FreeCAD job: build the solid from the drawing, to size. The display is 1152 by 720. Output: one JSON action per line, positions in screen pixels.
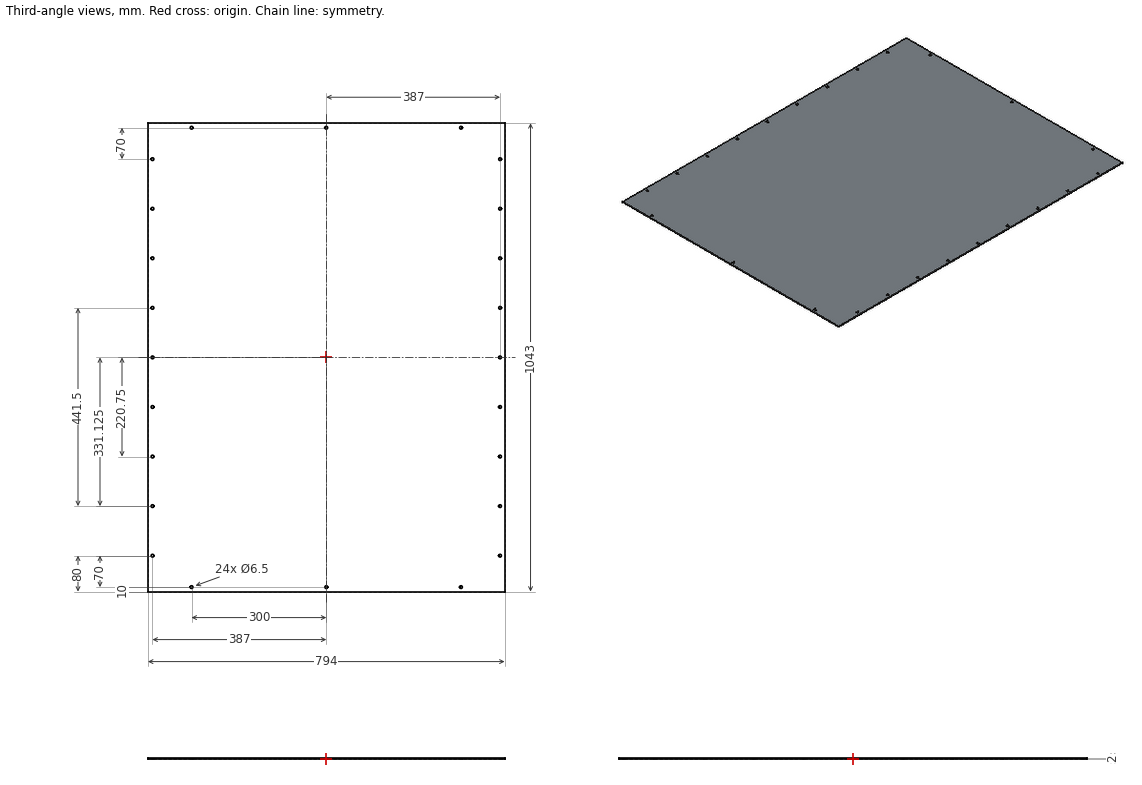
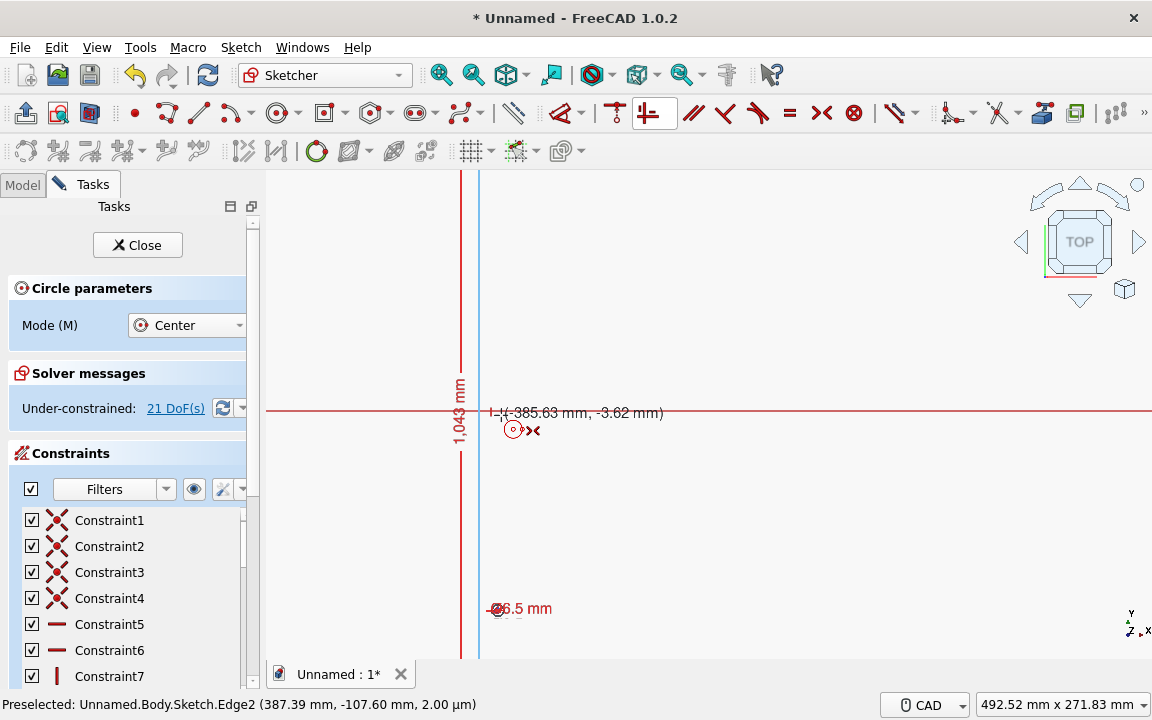
{"action": "left_click", "coordinate": [497, 411]}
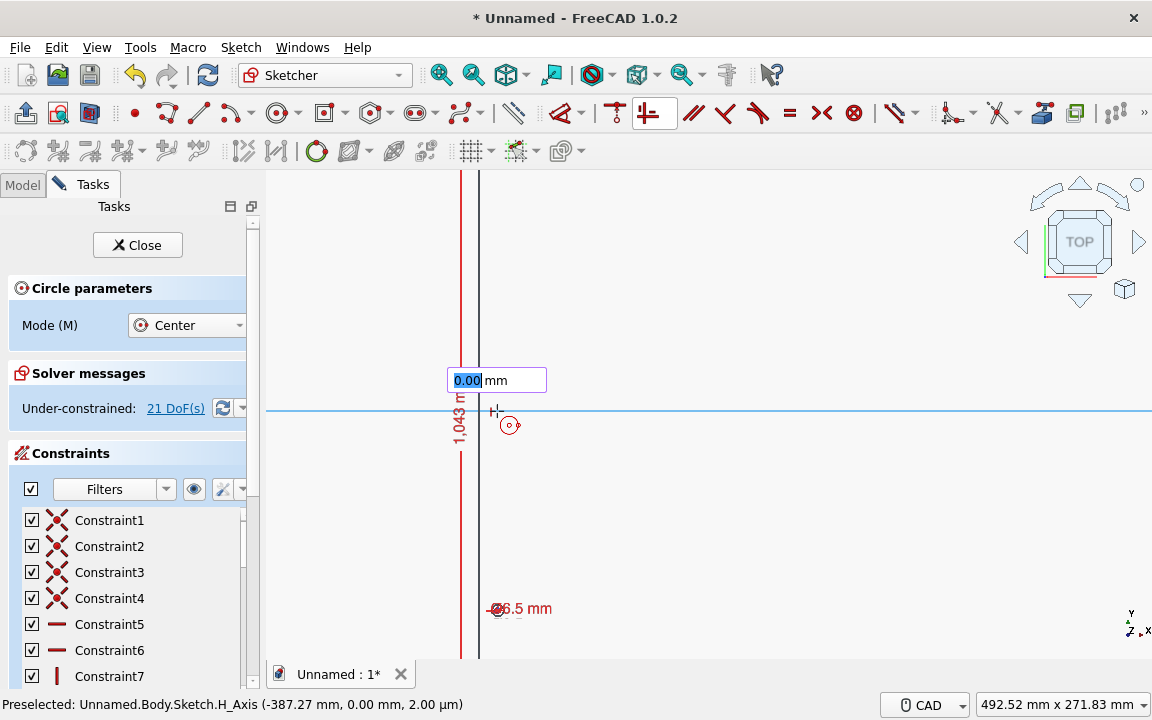
{"action": "scroll", "coordinate": [495, 417], "scroll_direction": "up", "scroll_amount": 6}
{"action": "mouse_move", "coordinate": [496, 416]}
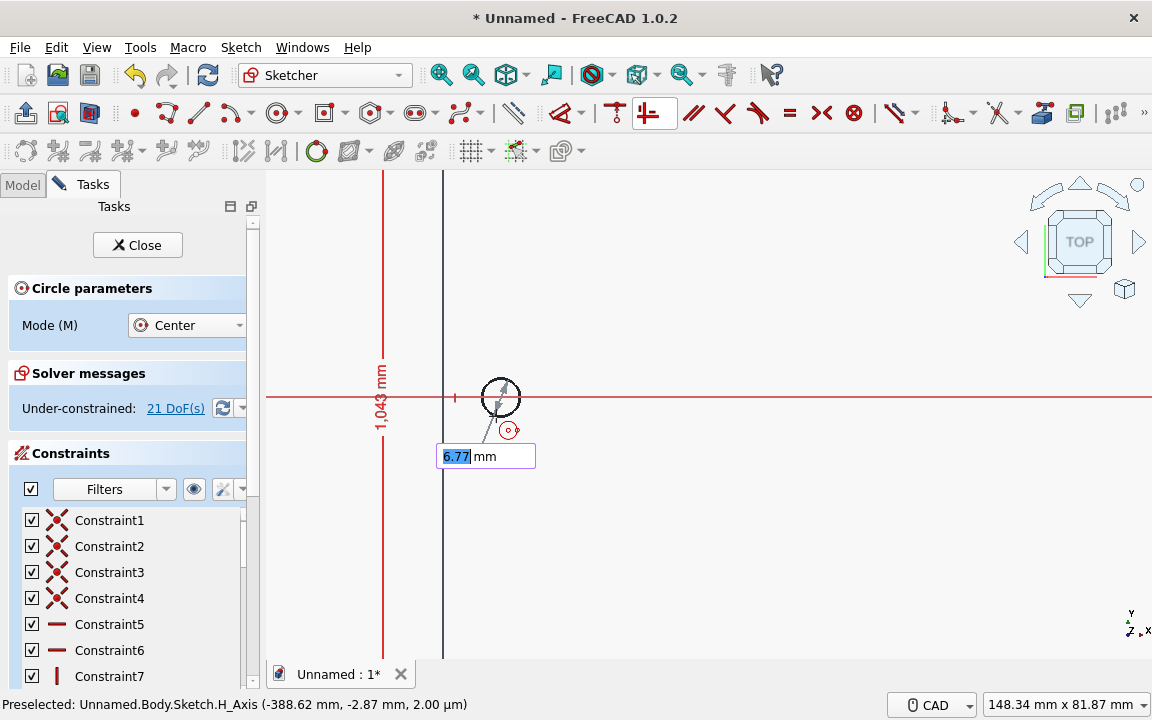
{"action": "type", "text": "6.5"}
{"action": "key", "text": "Return"}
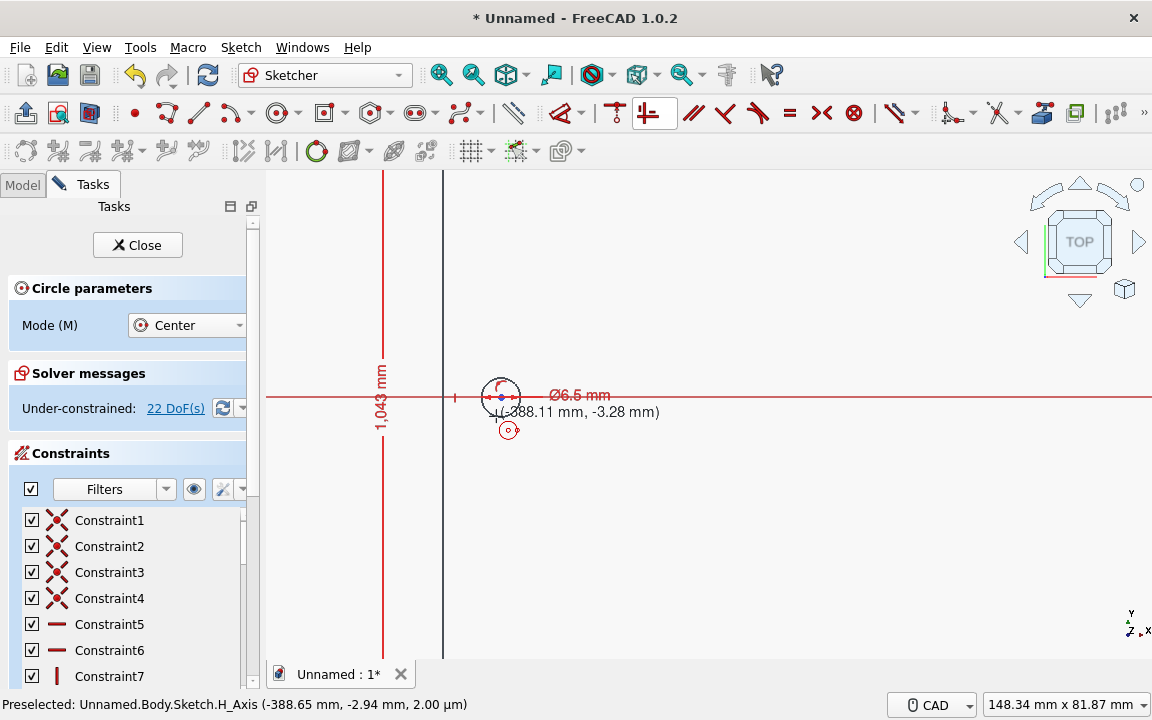
{"action": "scroll", "coordinate": [527, 415], "scroll_direction": "down", "scroll_amount": 15}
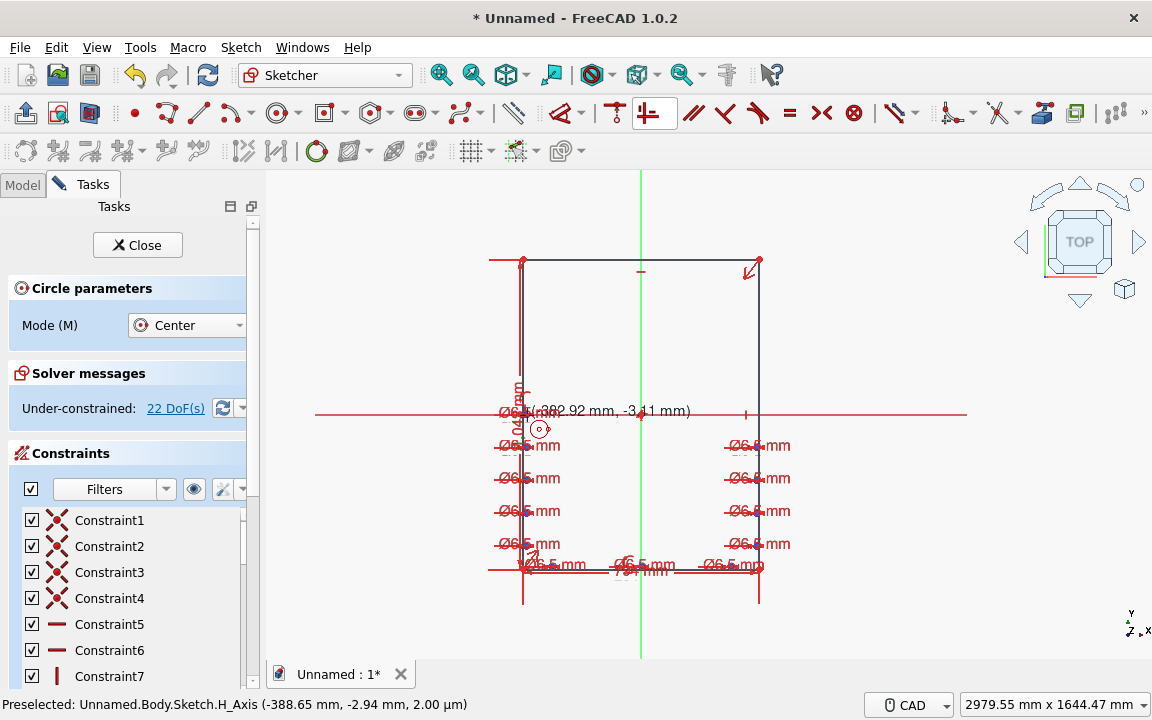
{"action": "scroll", "coordinate": [526, 382], "scroll_direction": "up", "scroll_amount": 16}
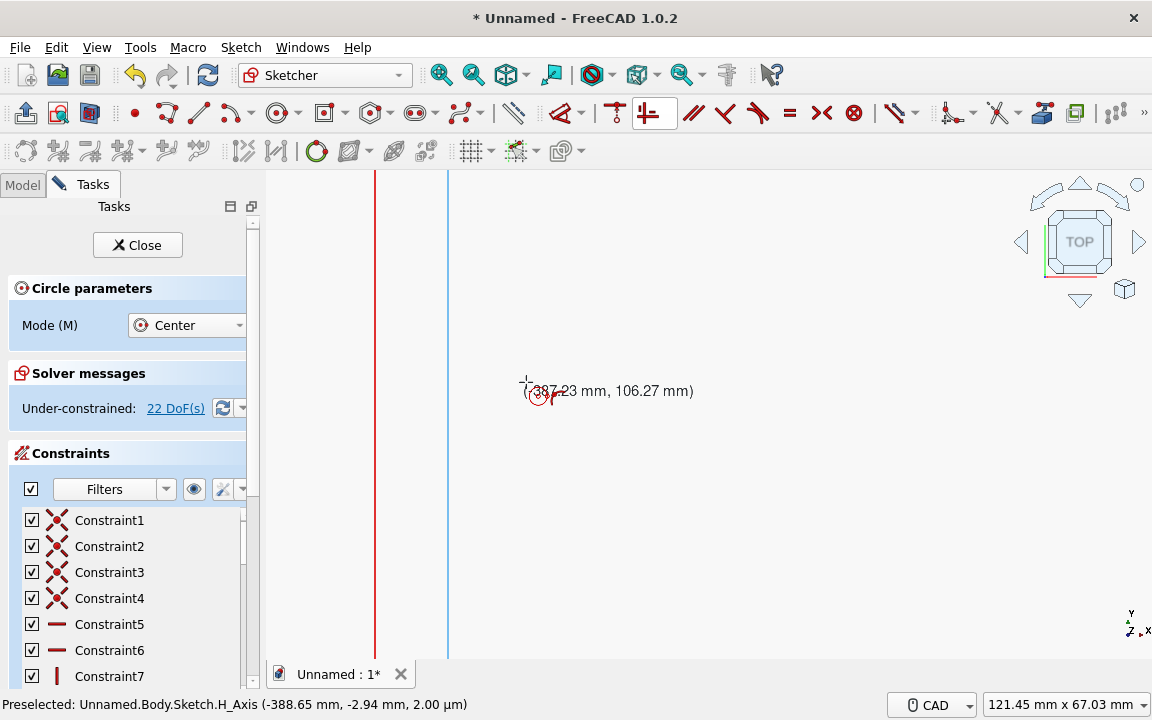
{"action": "scroll", "coordinate": [499, 375], "scroll_direction": "down", "scroll_amount": 15}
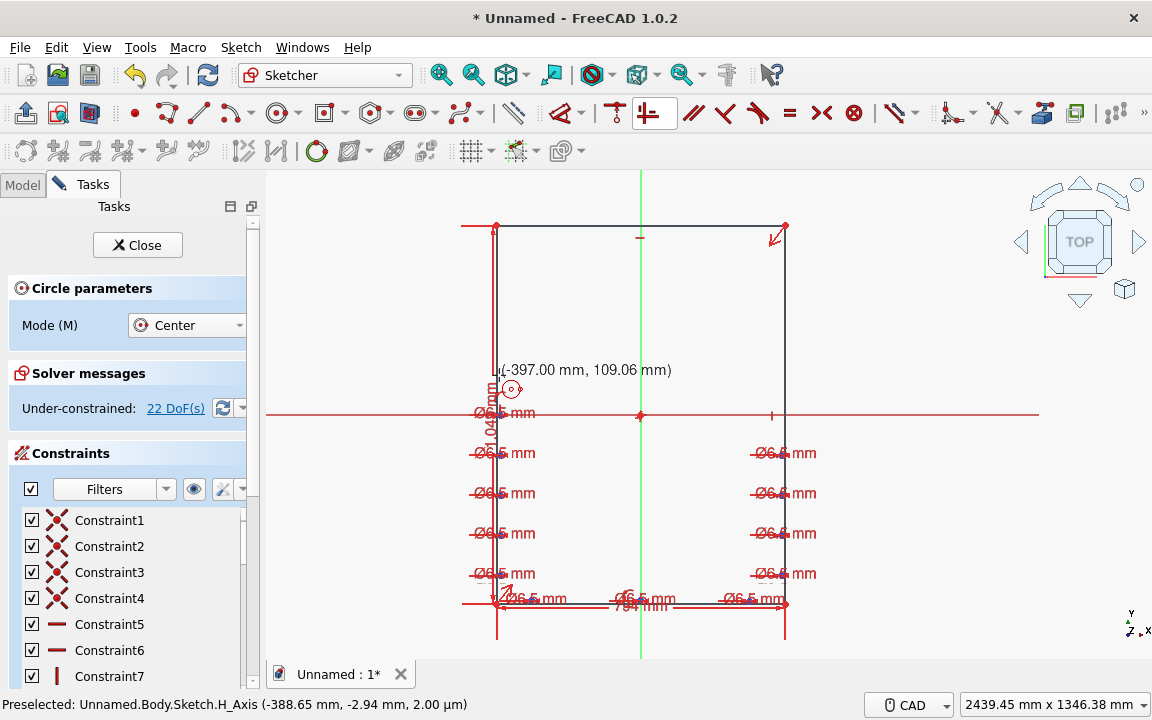
{"action": "scroll", "coordinate": [500, 375], "scroll_direction": "up", "scroll_amount": 8}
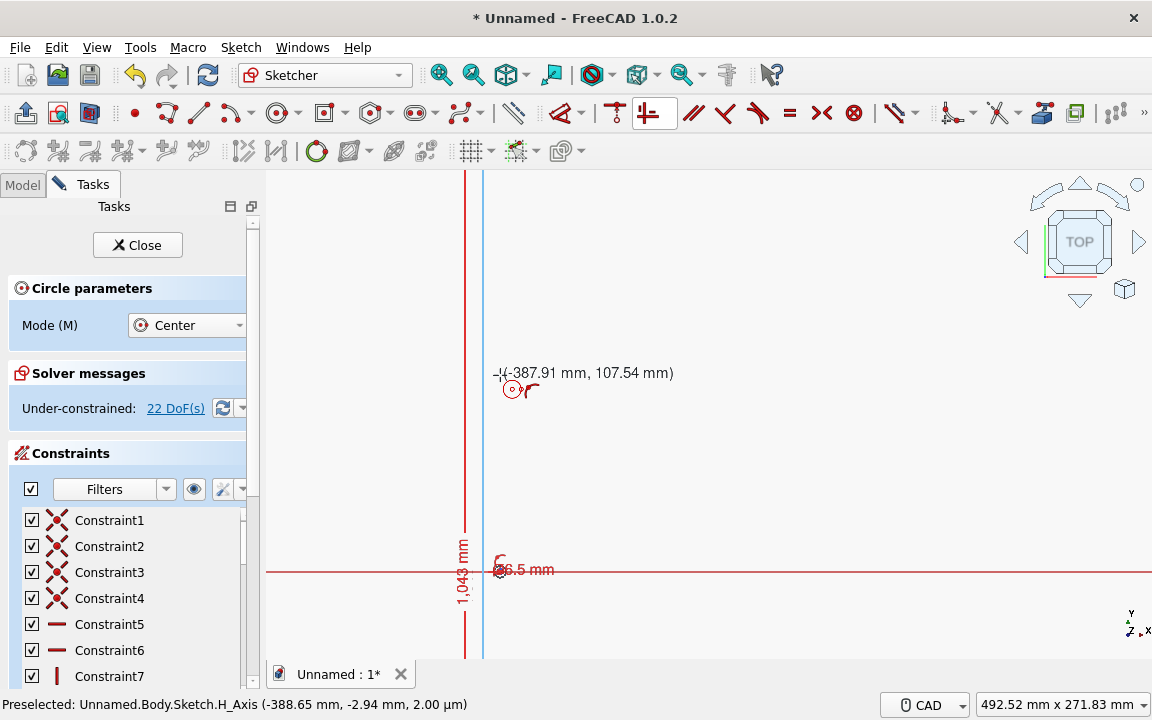
{"action": "left_click", "coordinate": [501, 373]}
{"action": "mouse_move", "coordinate": [505, 369]}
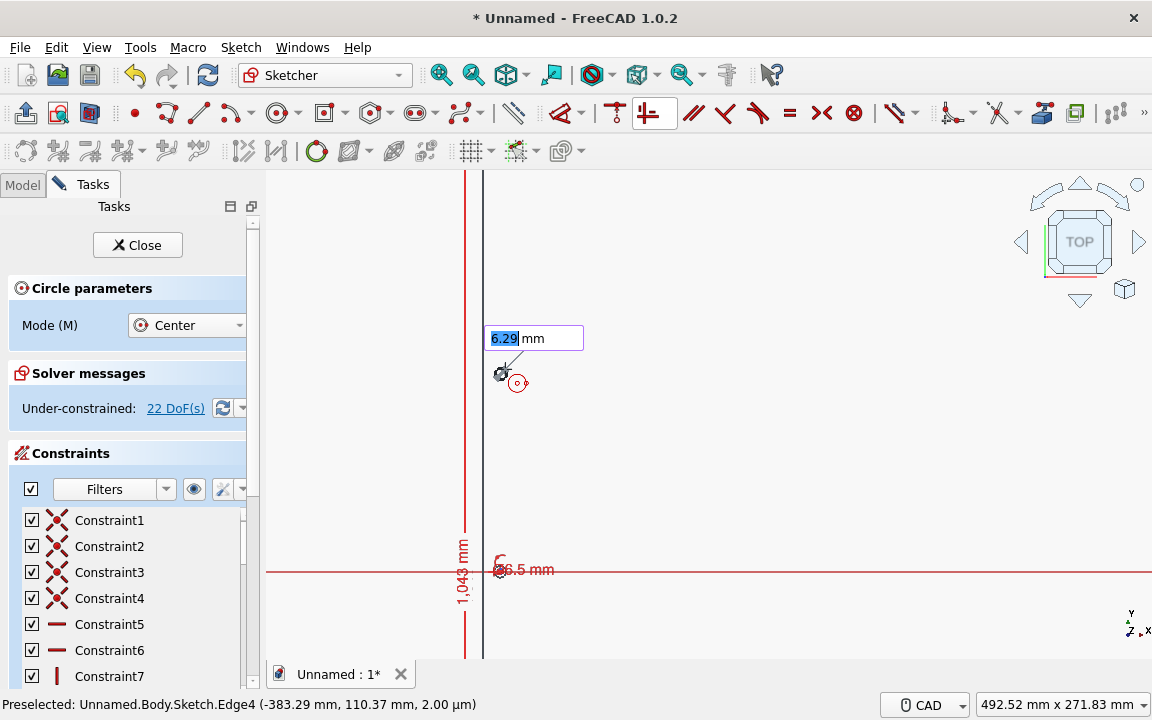
{"action": "type", "text": "6.5"}
{"action": "key", "text": "Return"}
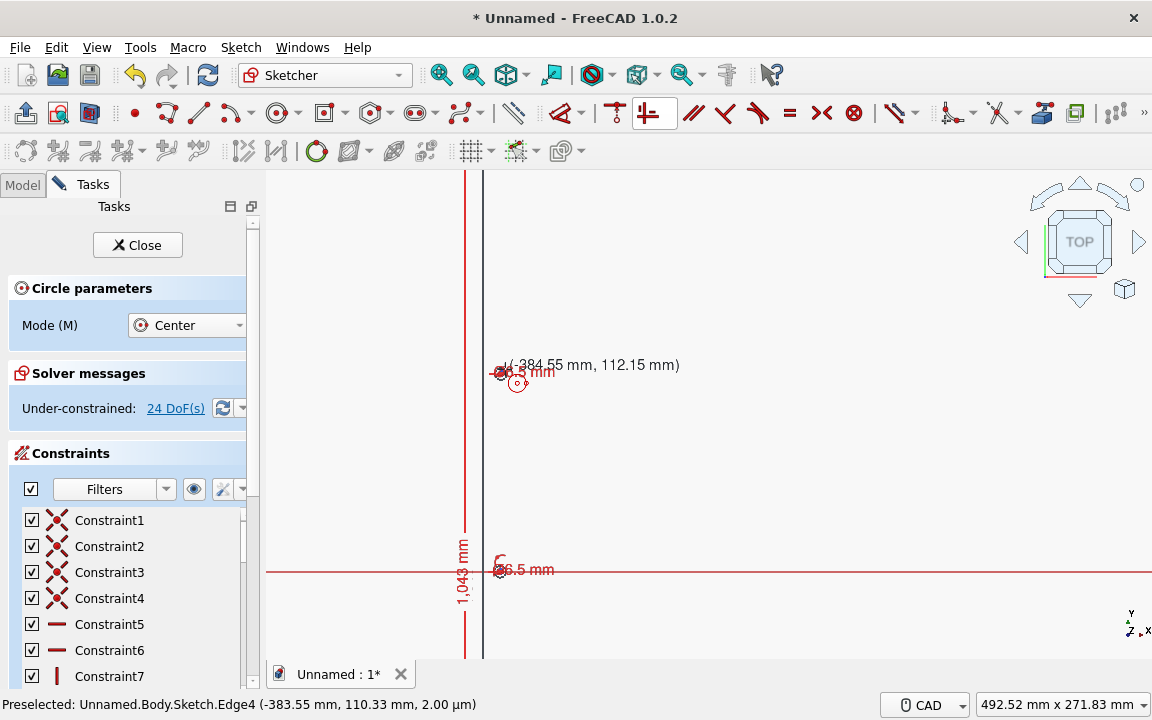
{"action": "scroll", "coordinate": [530, 383], "scroll_direction": "down", "scroll_amount": 9}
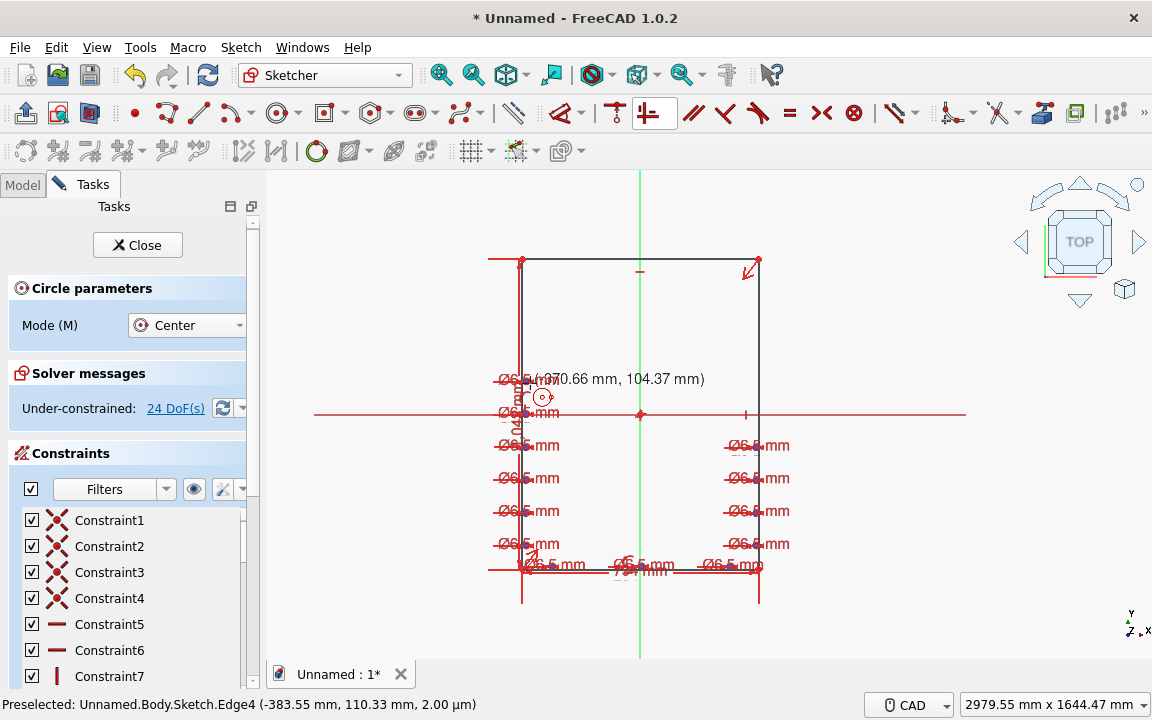
{"action": "scroll", "coordinate": [525, 349], "scroll_direction": "up", "scroll_amount": 16}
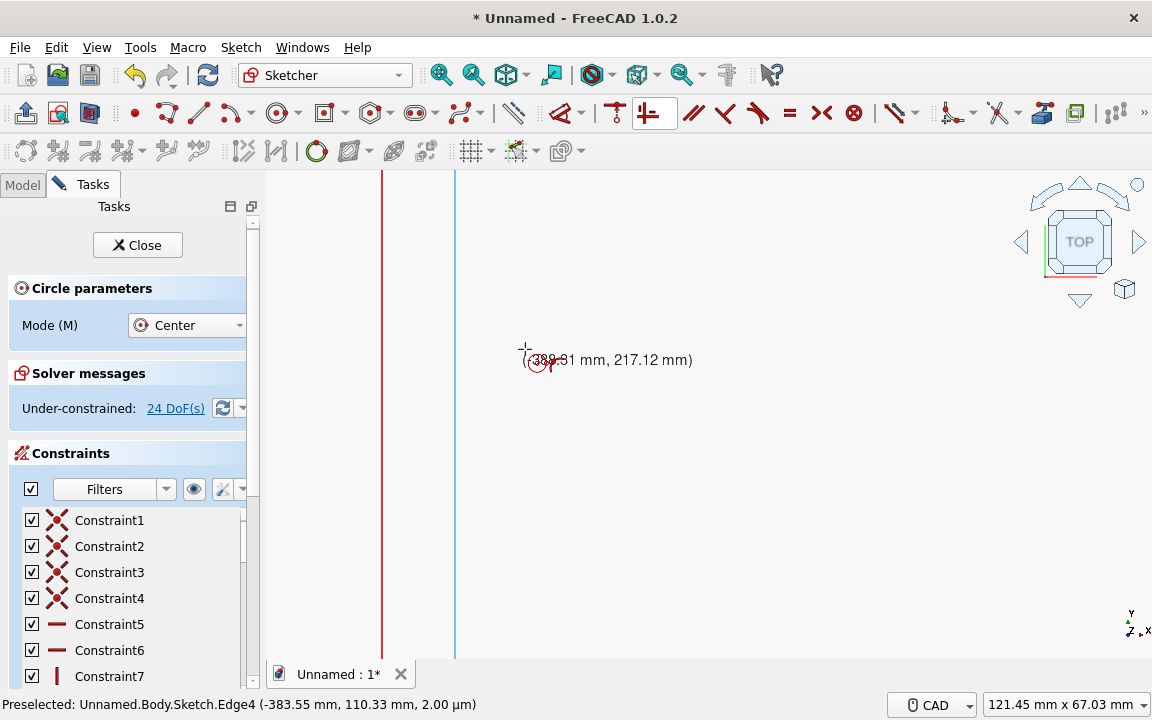
{"action": "scroll", "coordinate": [498, 334], "scroll_direction": "down", "scroll_amount": 15}